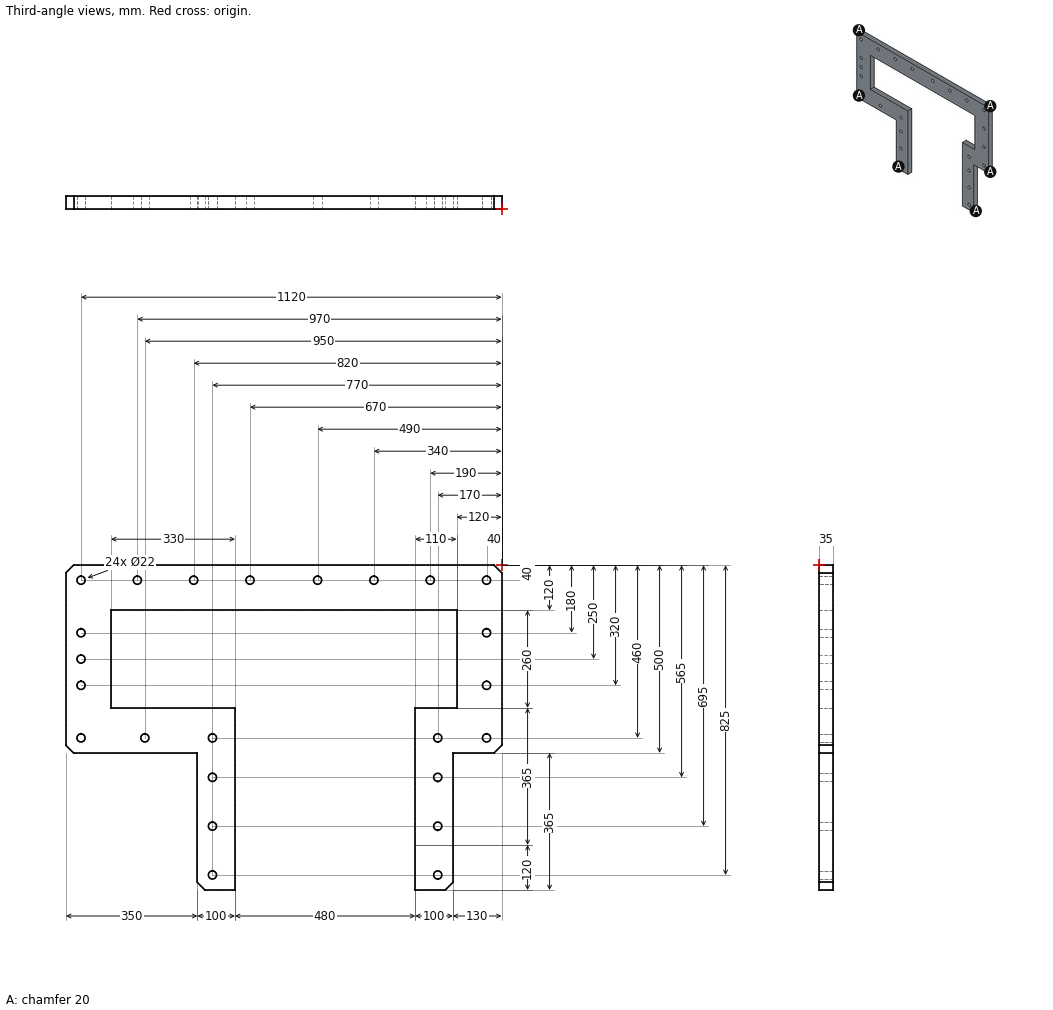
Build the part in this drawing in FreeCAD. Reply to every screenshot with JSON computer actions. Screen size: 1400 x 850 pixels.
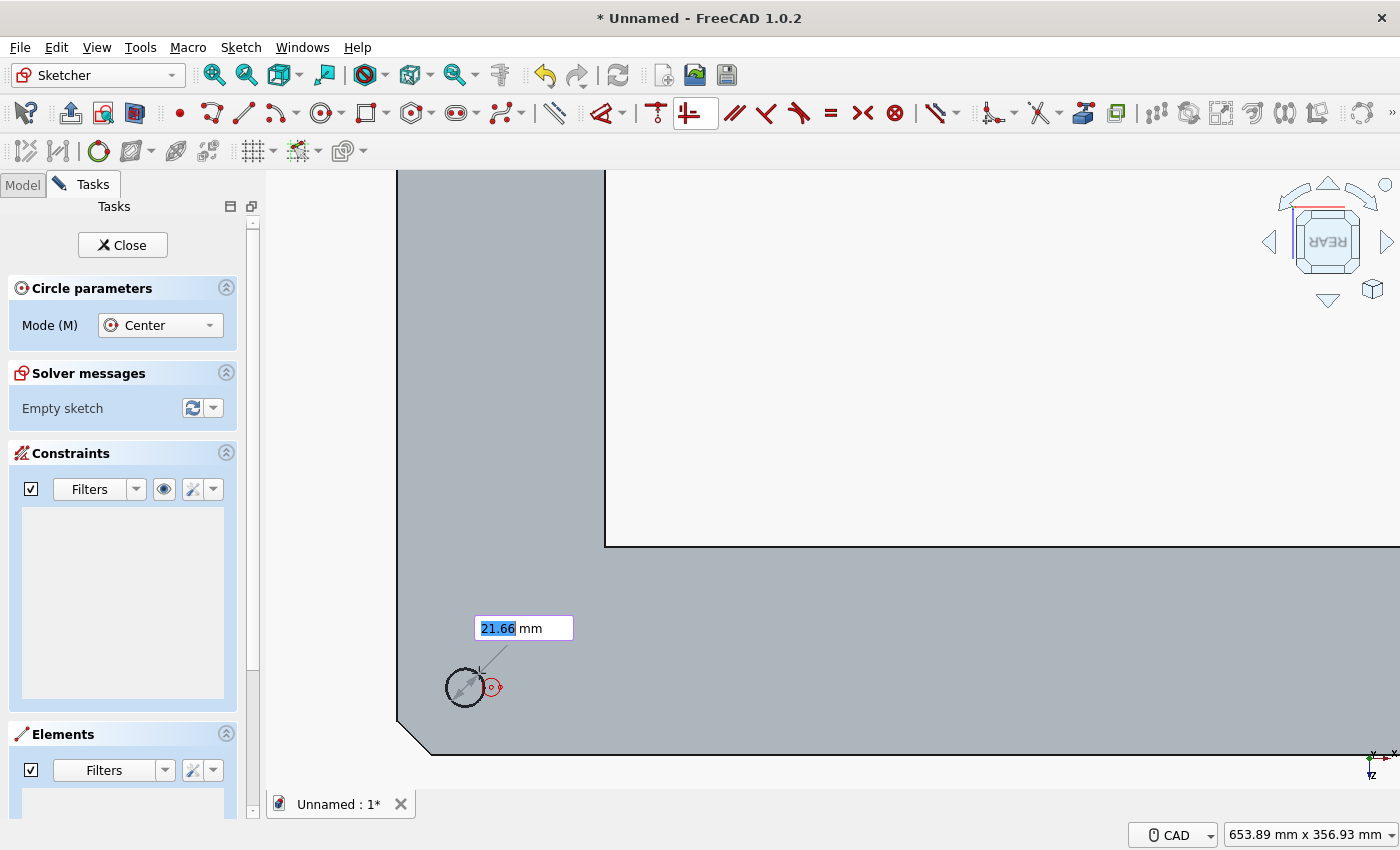
{"action": "left_click", "coordinate": [480, 672]}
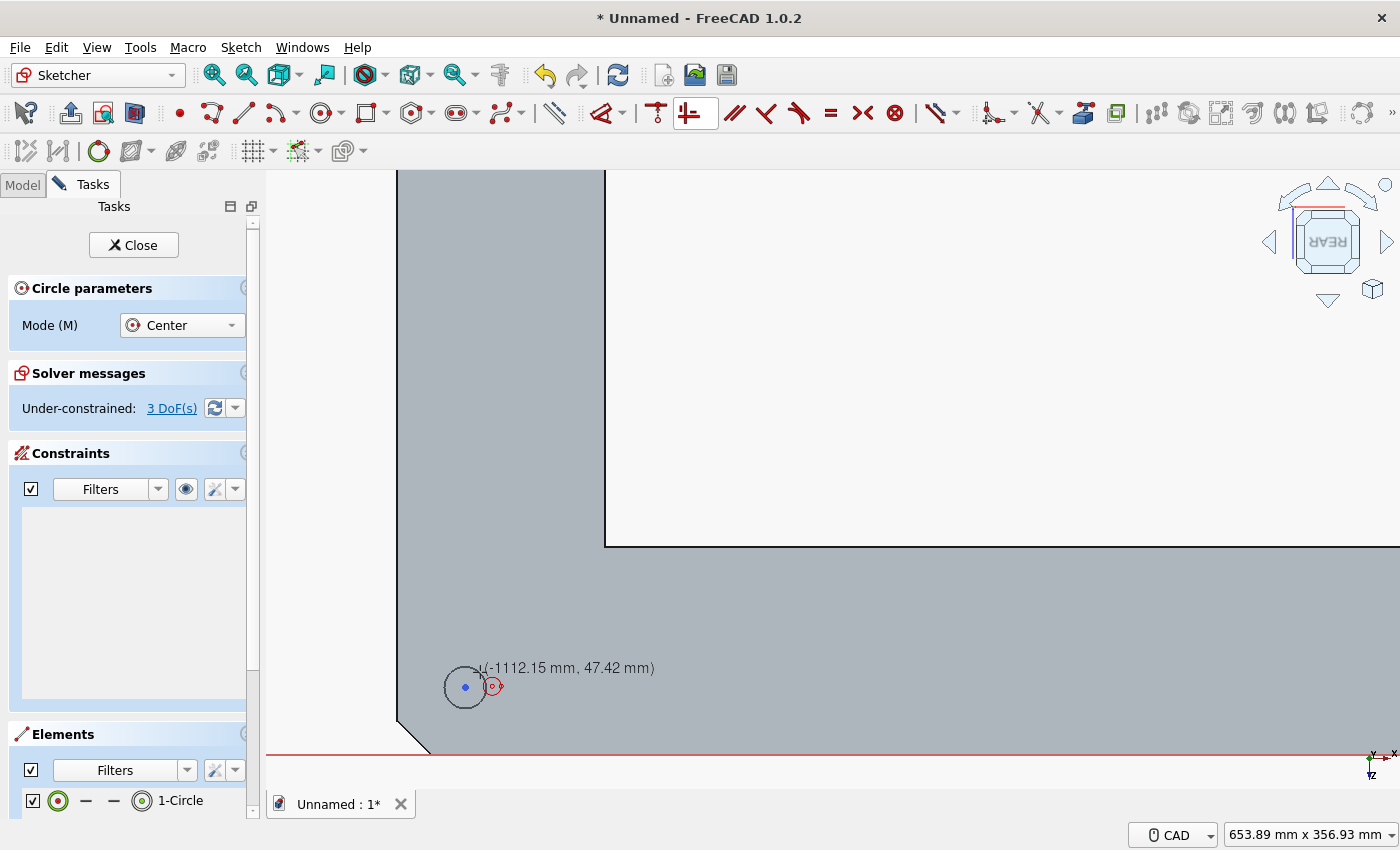
{"action": "scroll", "coordinate": [479, 673], "scroll_direction": "down", "scroll_amount": 6}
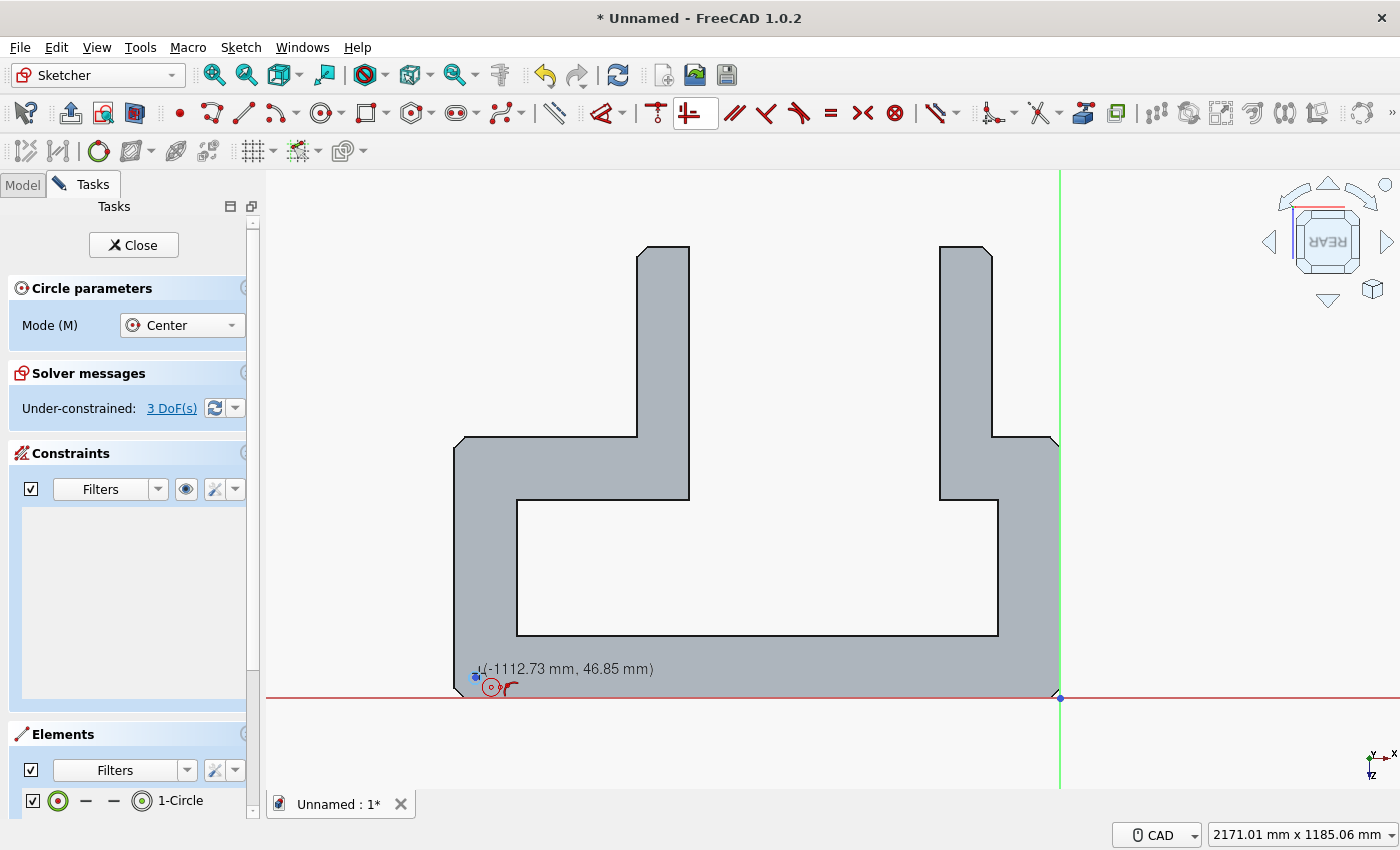
{"action": "left_click", "coordinate": [554, 677]}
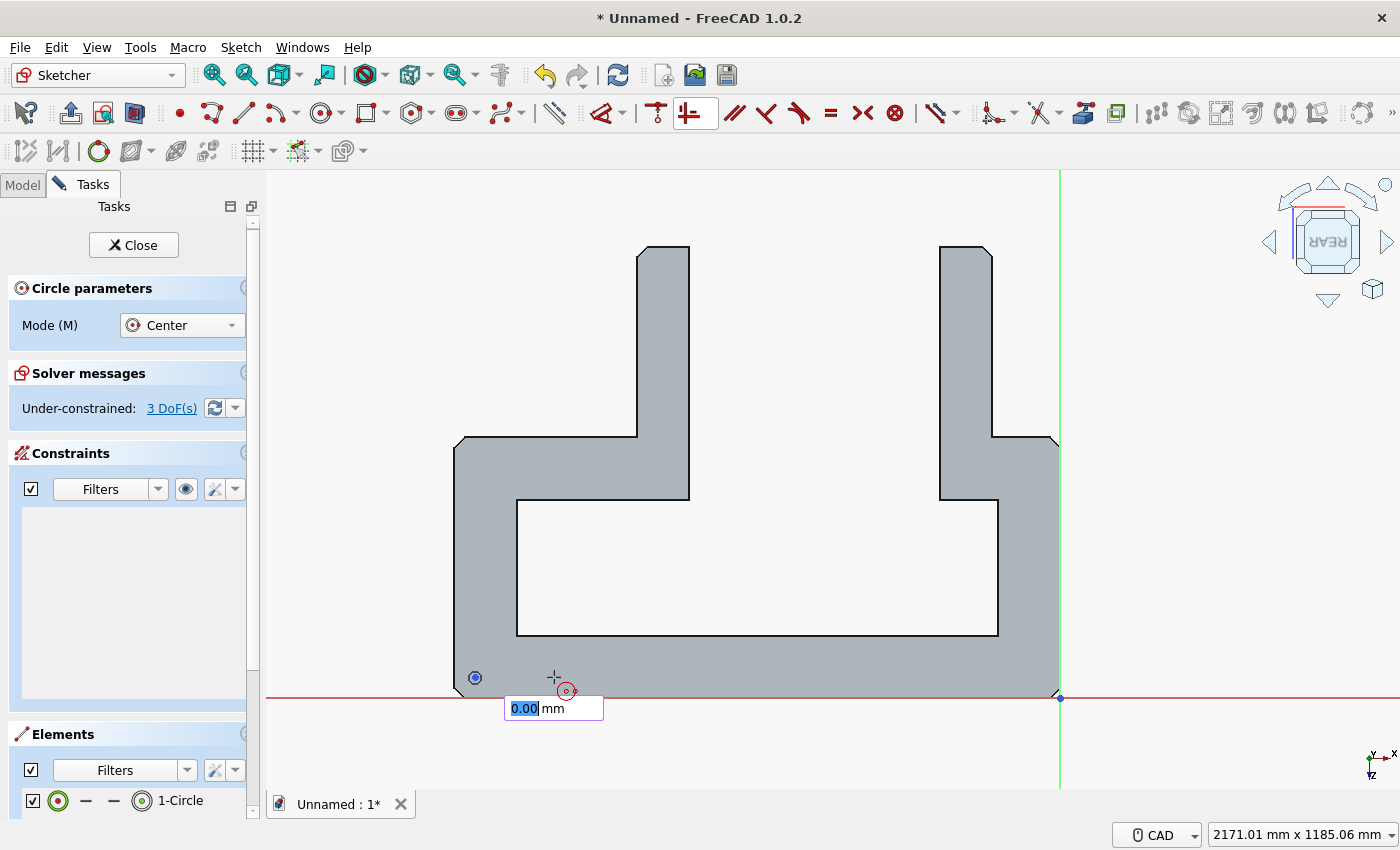
{"action": "scroll", "coordinate": [558, 673], "scroll_direction": "up", "scroll_amount": 6}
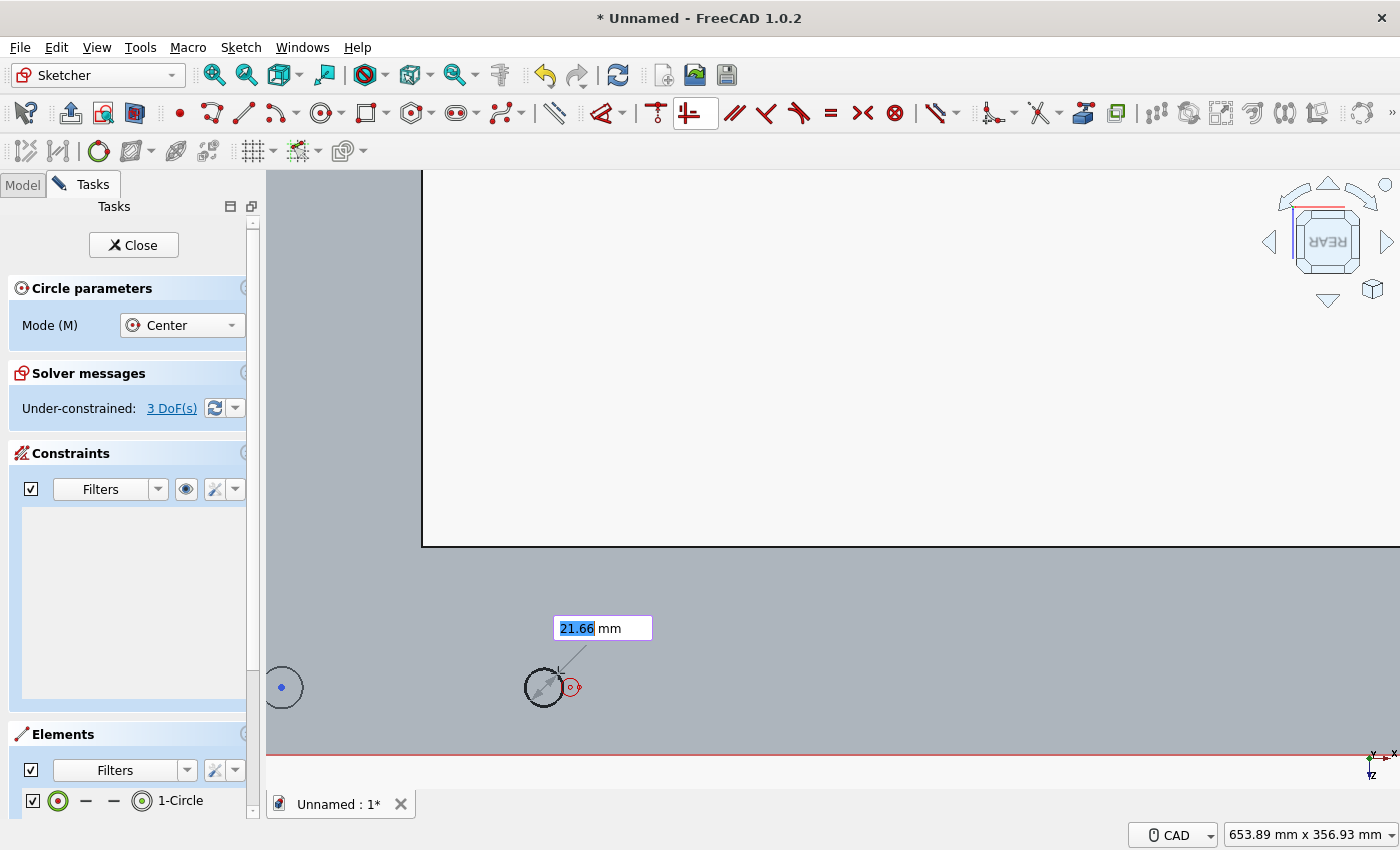
{"action": "left_click", "coordinate": [557, 672]}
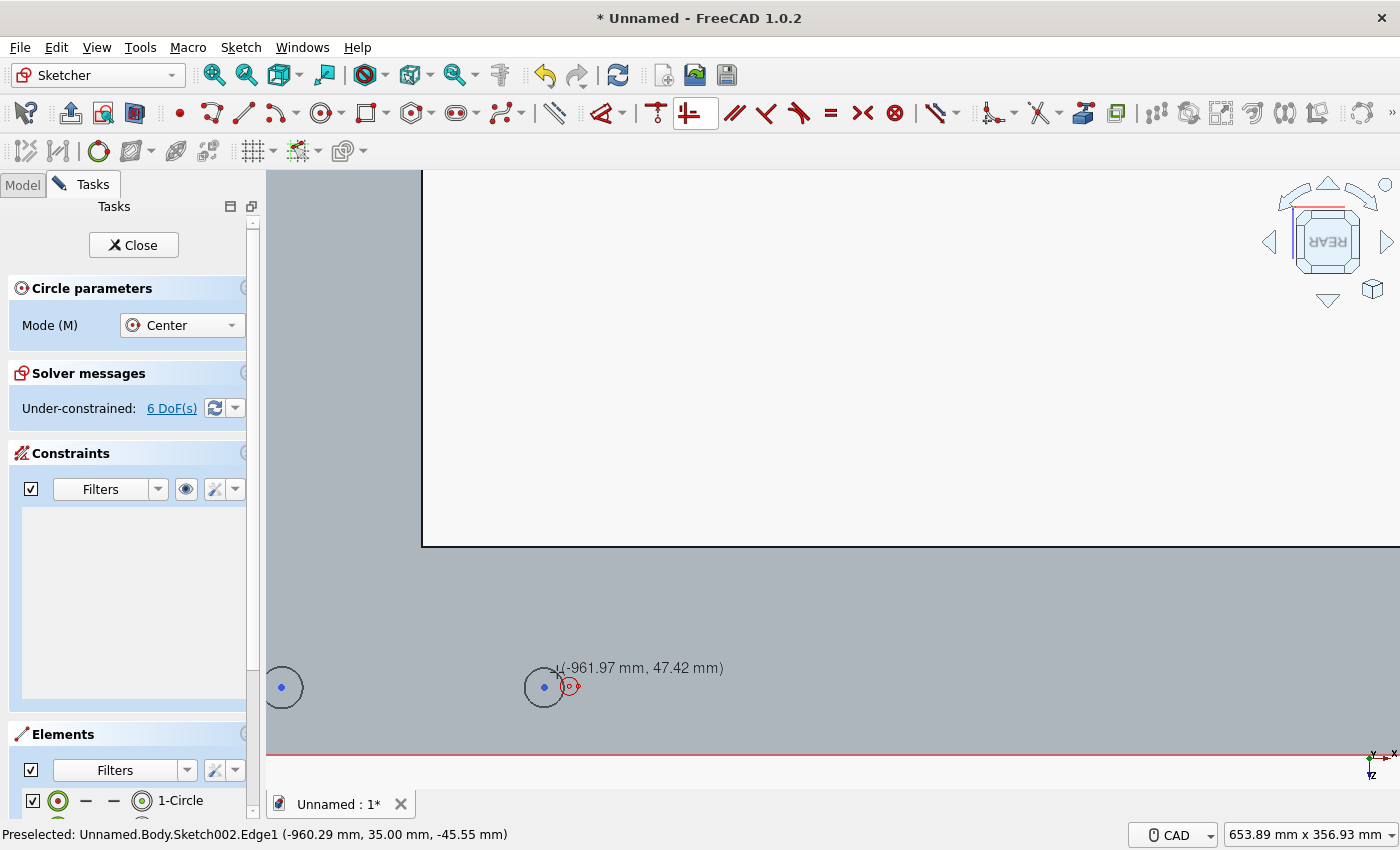
{"action": "scroll", "coordinate": [558, 673], "scroll_direction": "down", "scroll_amount": 6}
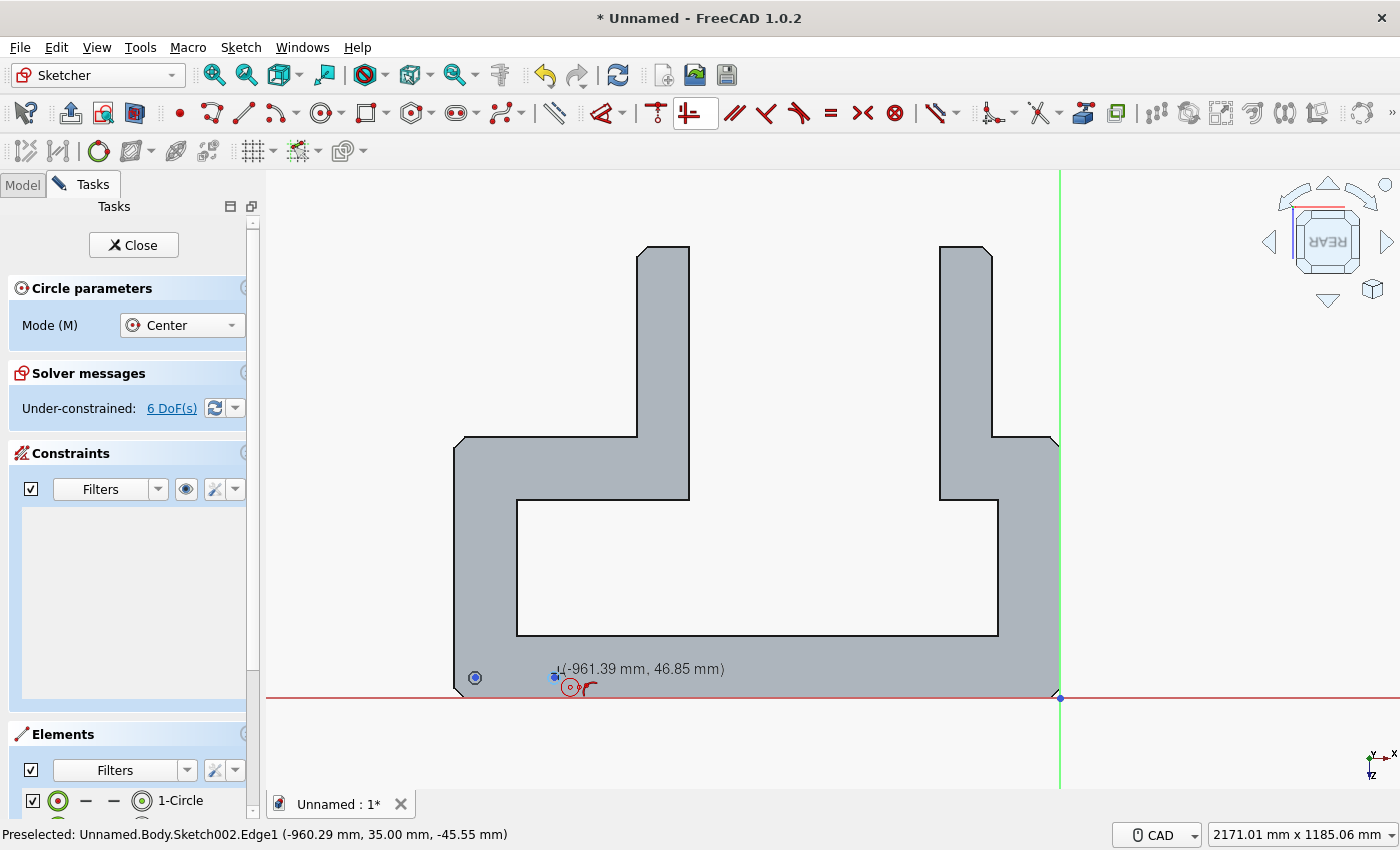
{"action": "left_click", "coordinate": [632, 677]}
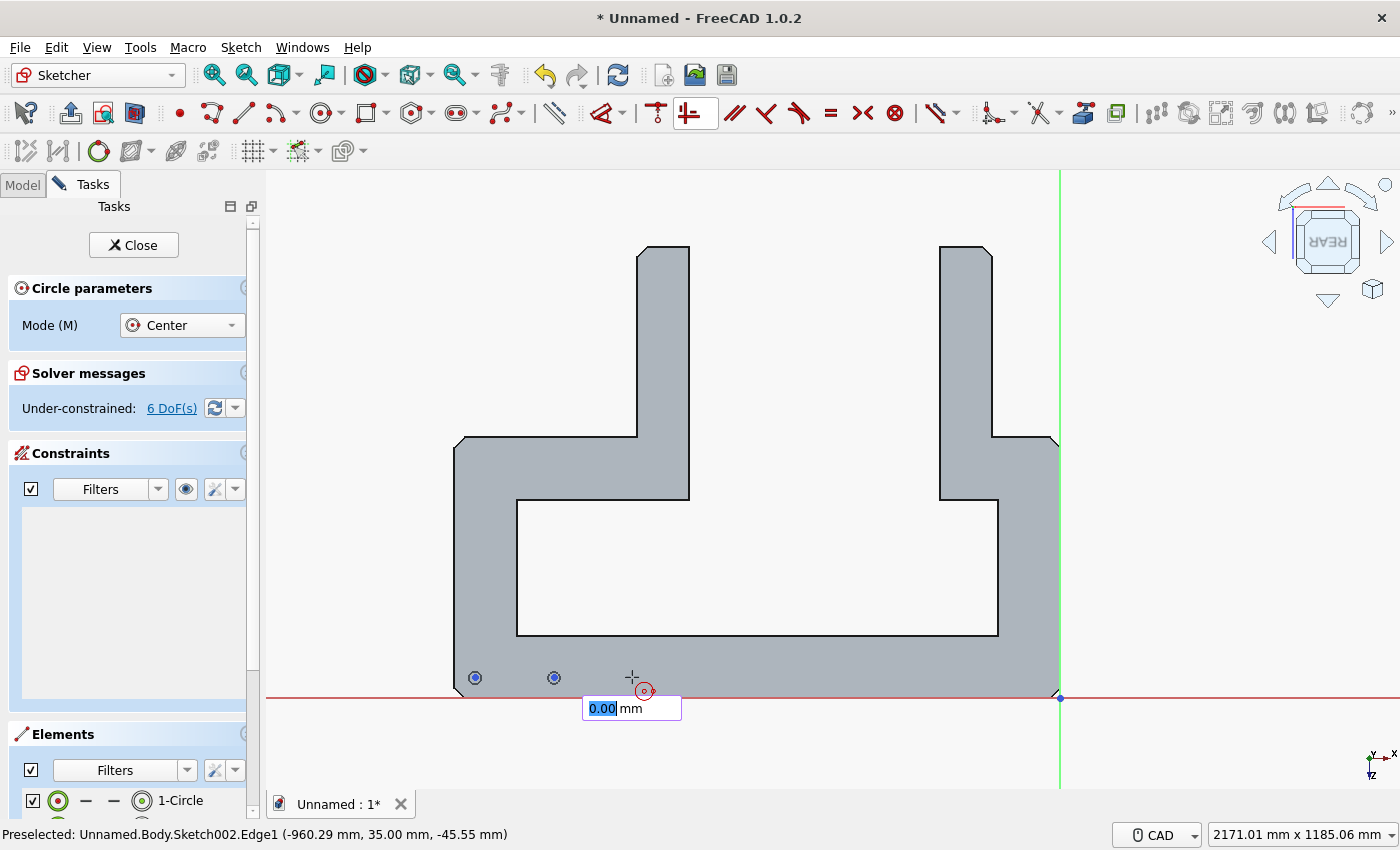
{"action": "scroll", "coordinate": [636, 673], "scroll_direction": "up", "scroll_amount": 6}